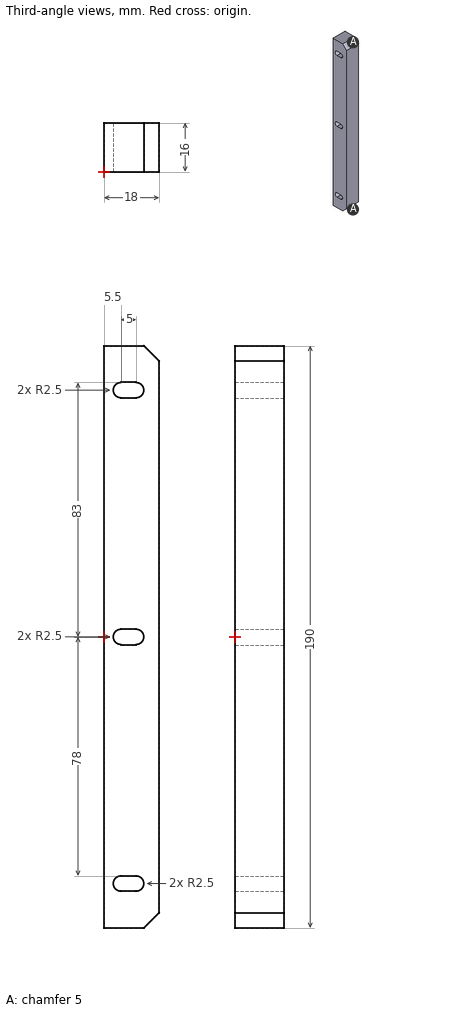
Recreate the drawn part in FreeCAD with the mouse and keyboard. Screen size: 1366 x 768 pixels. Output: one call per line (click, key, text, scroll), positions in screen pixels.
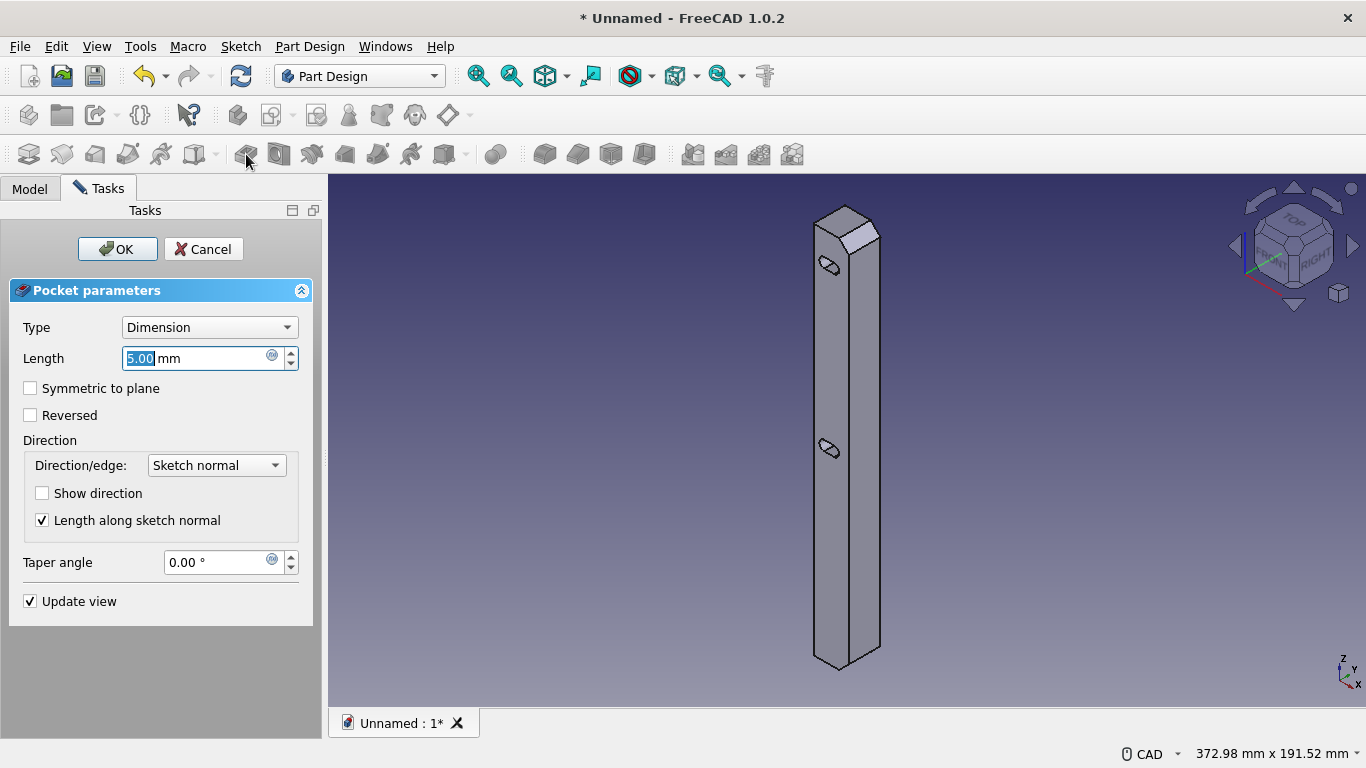
click(210, 328)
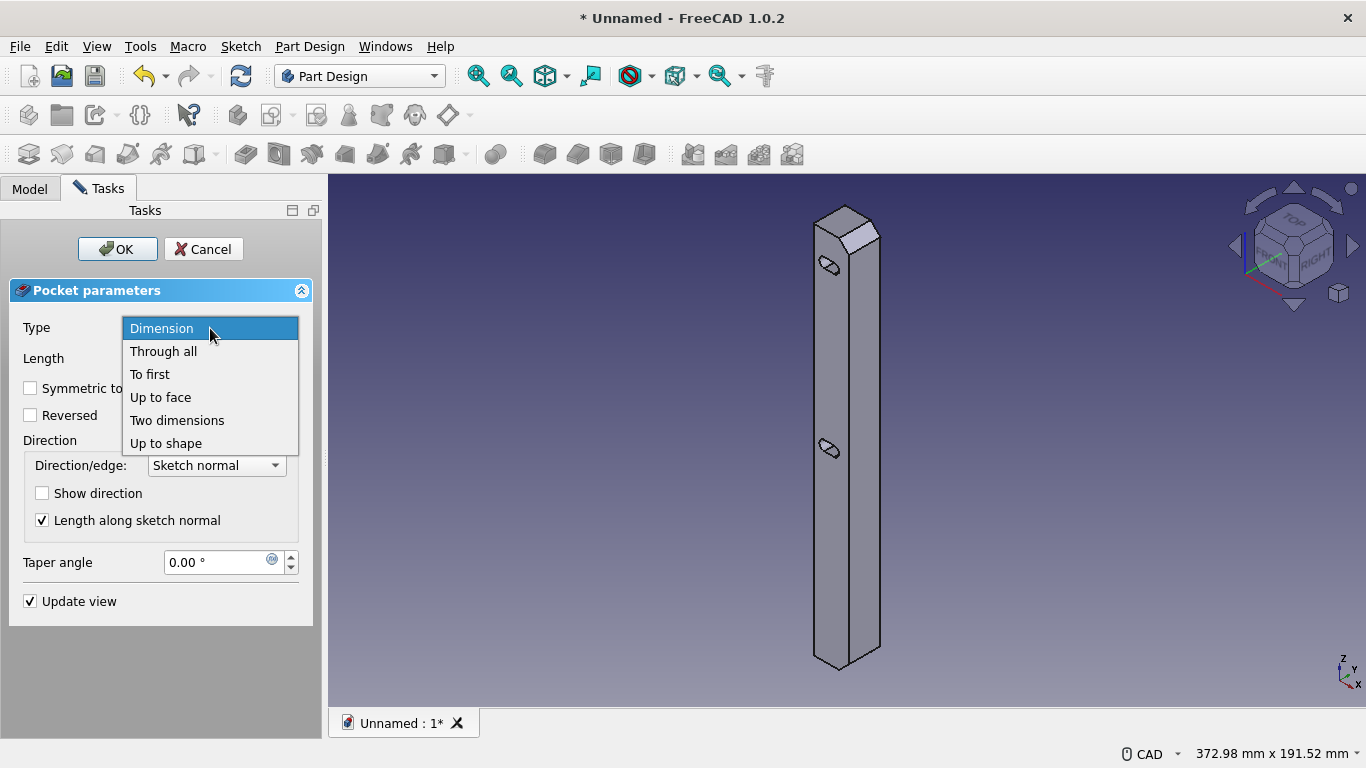
click(208, 374)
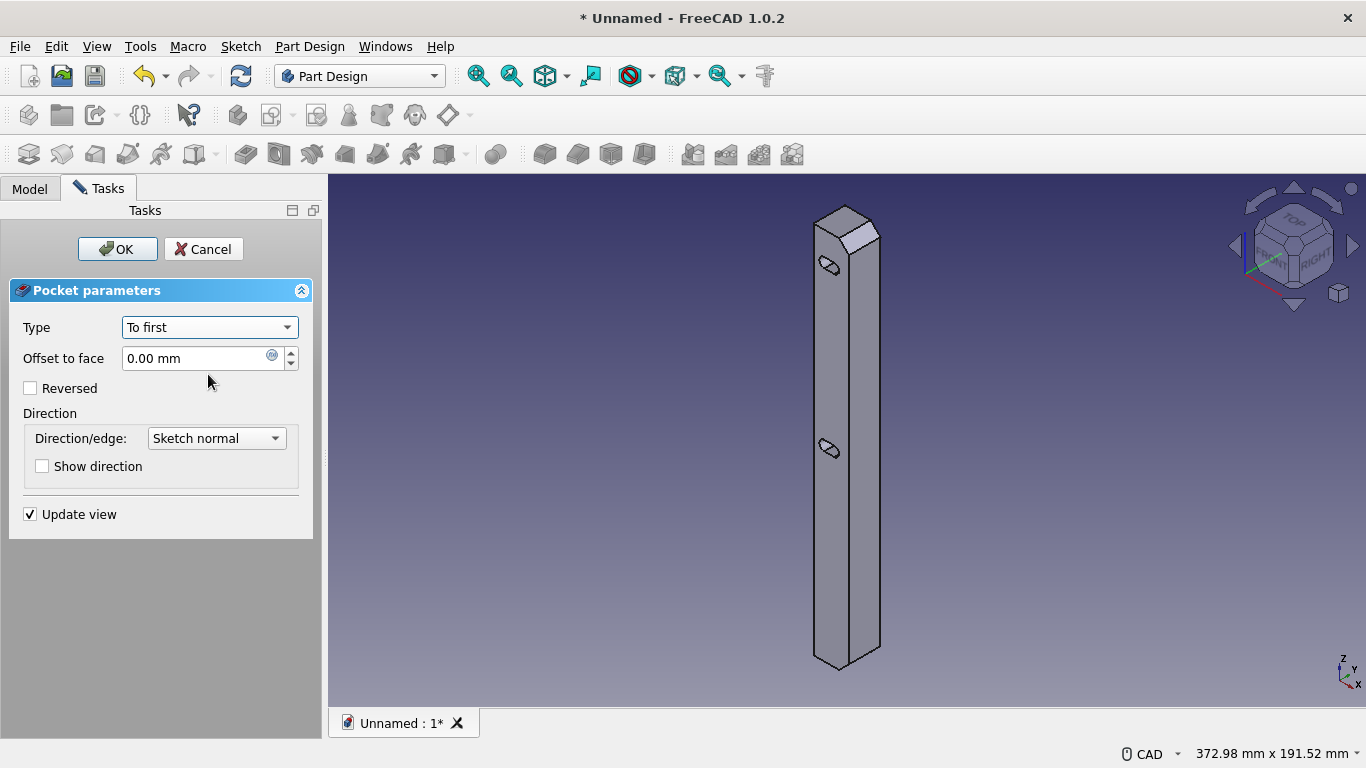
click(118, 249)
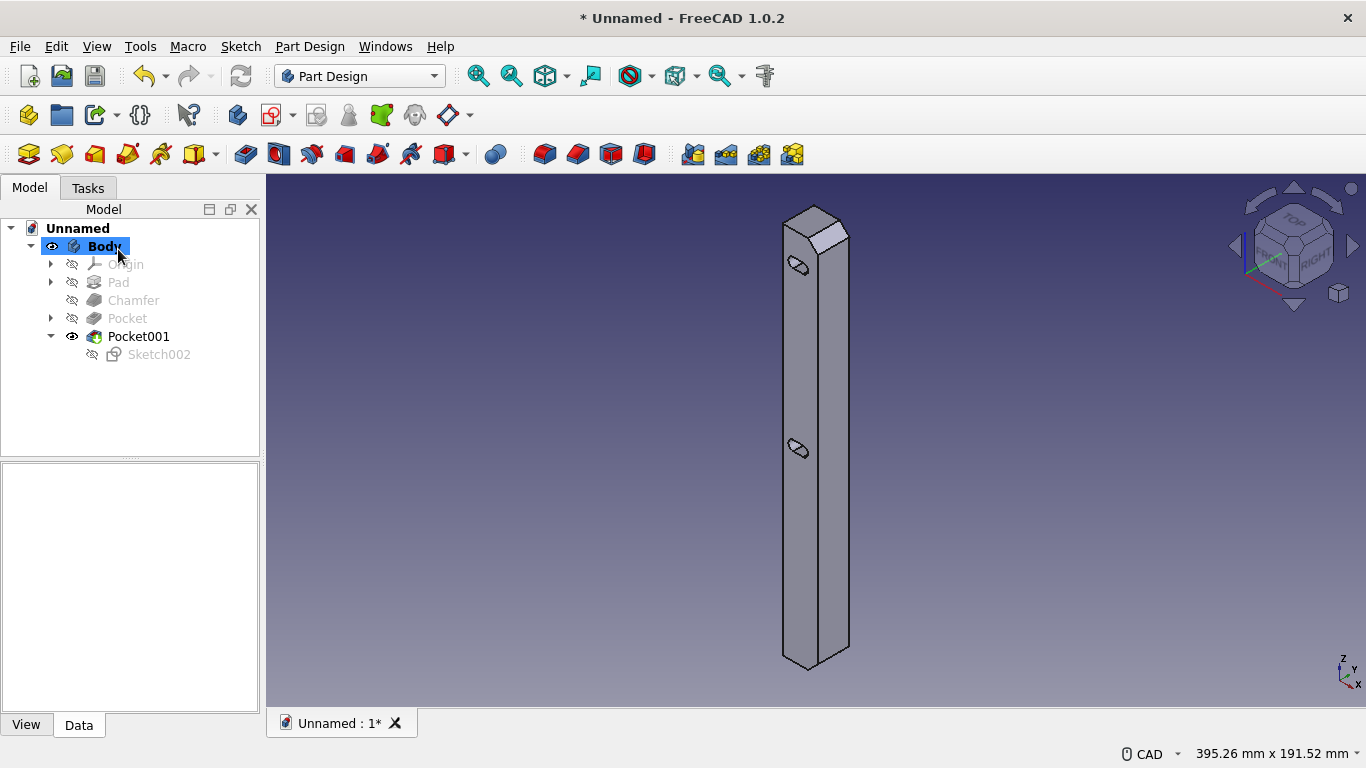
click(800, 325)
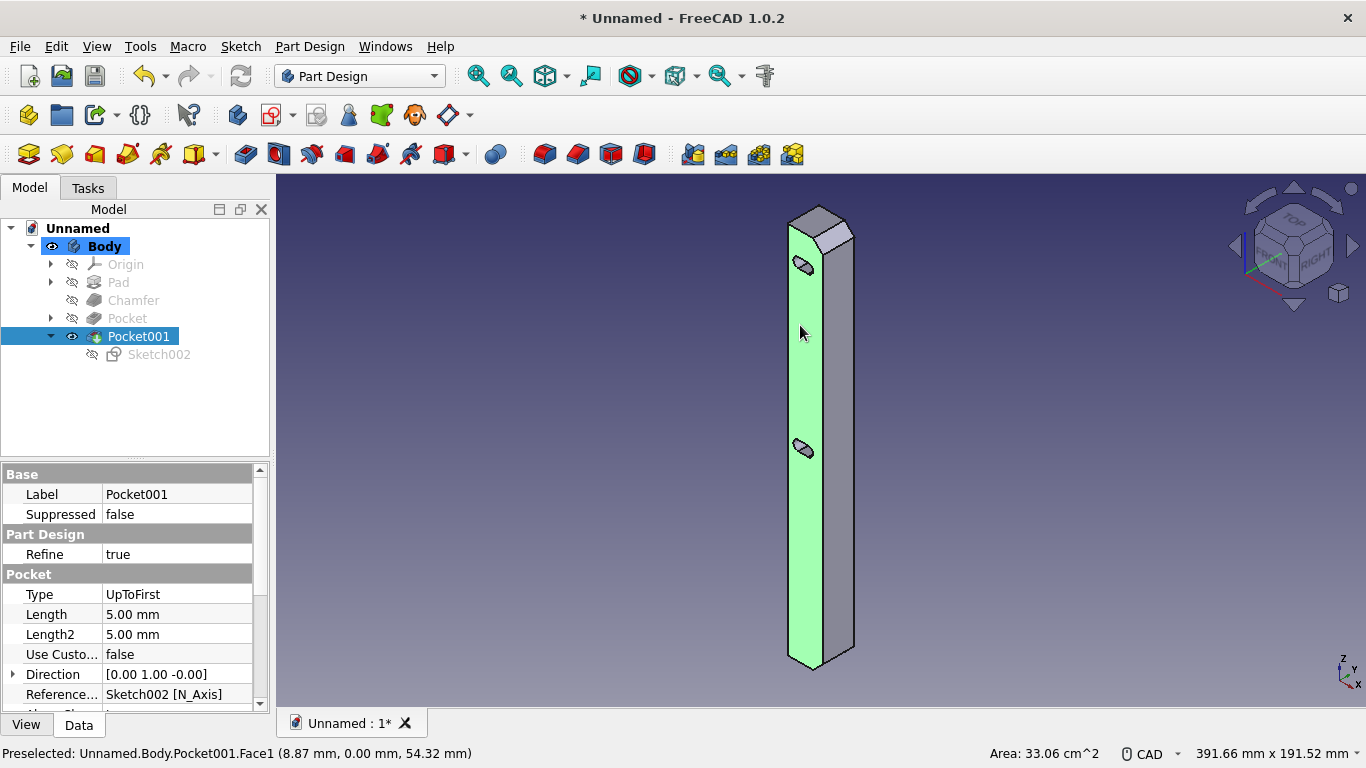
click(270, 116)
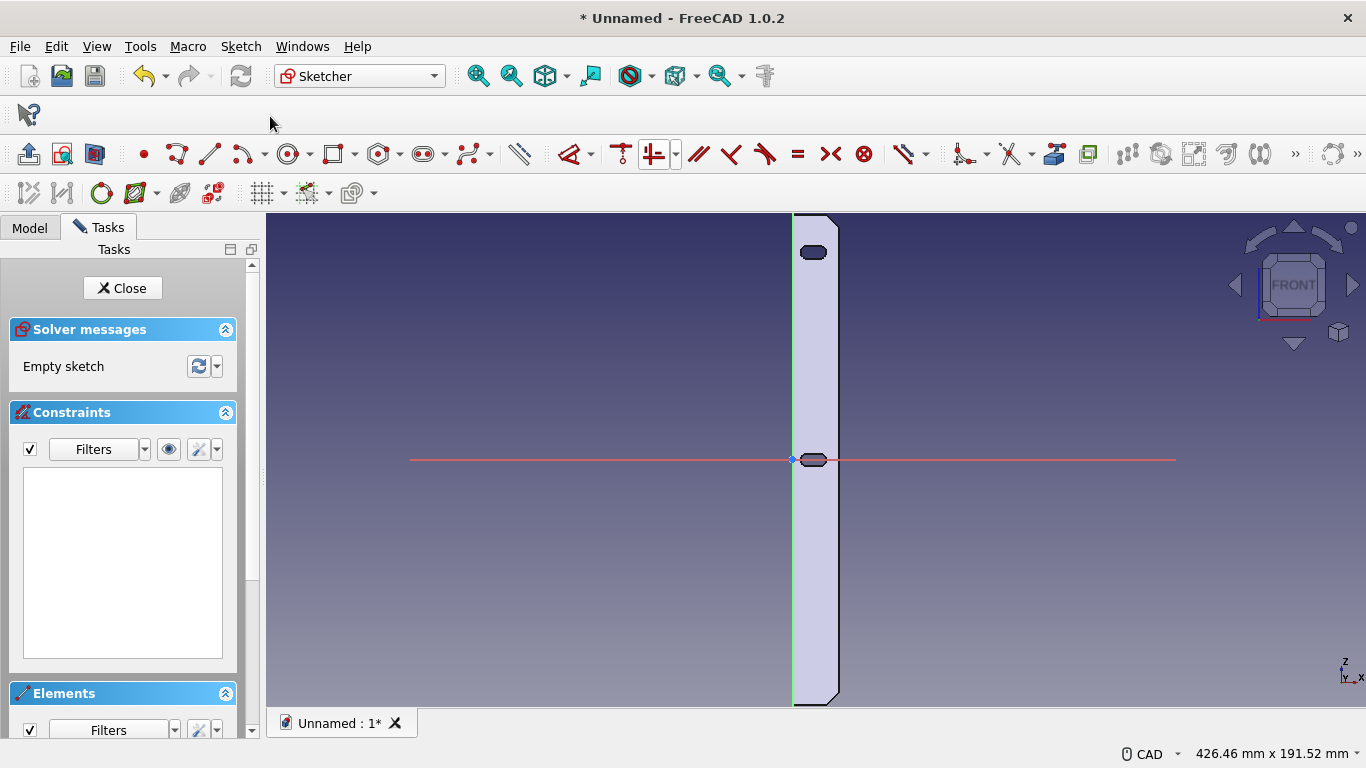
scroll(817, 679, up, 15)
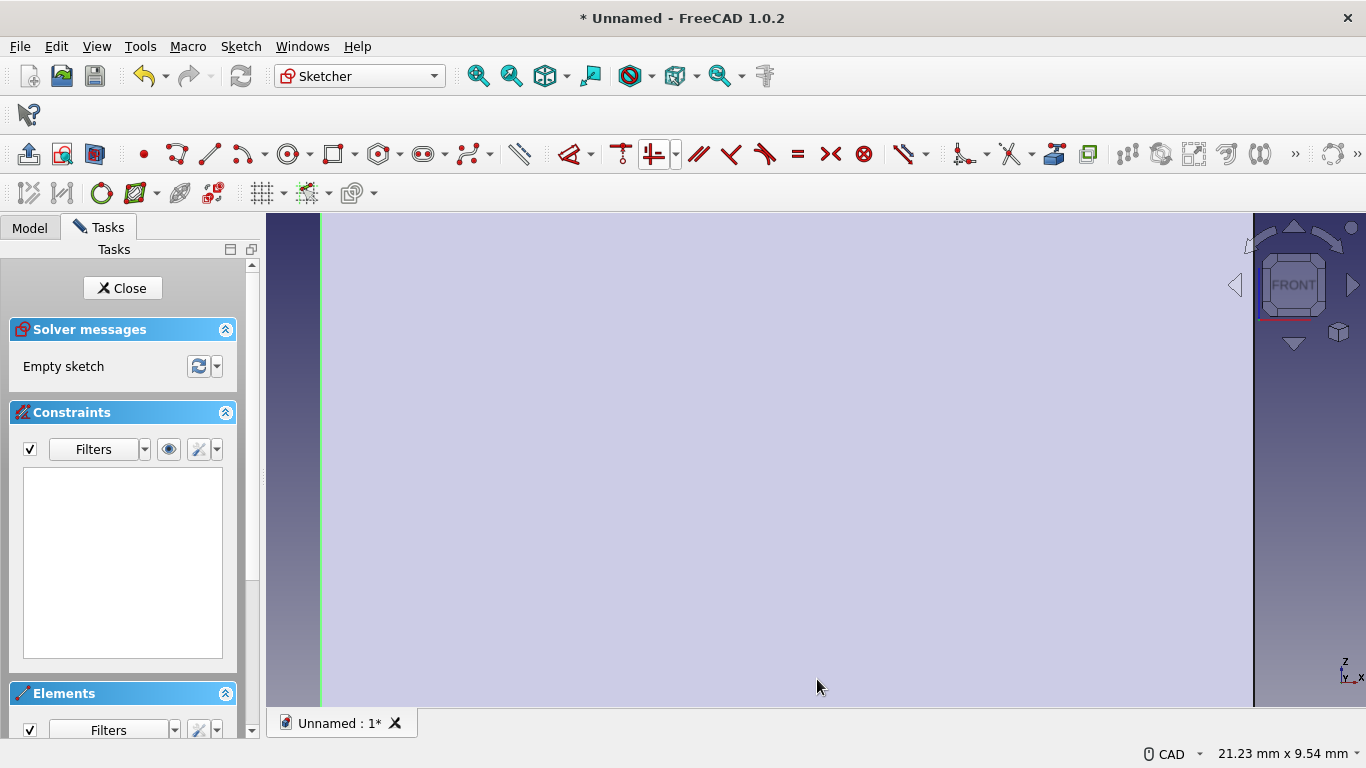
key(g)
key(s)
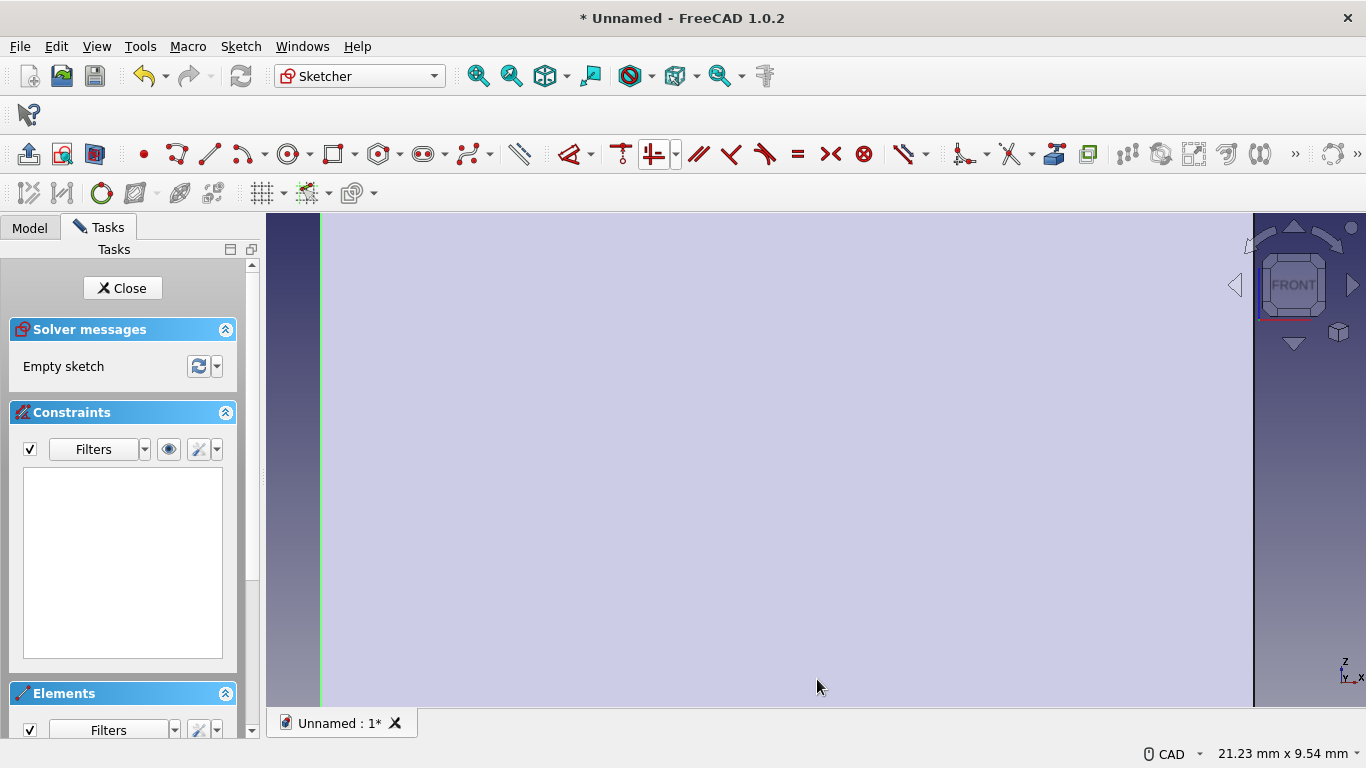
click(606, 433)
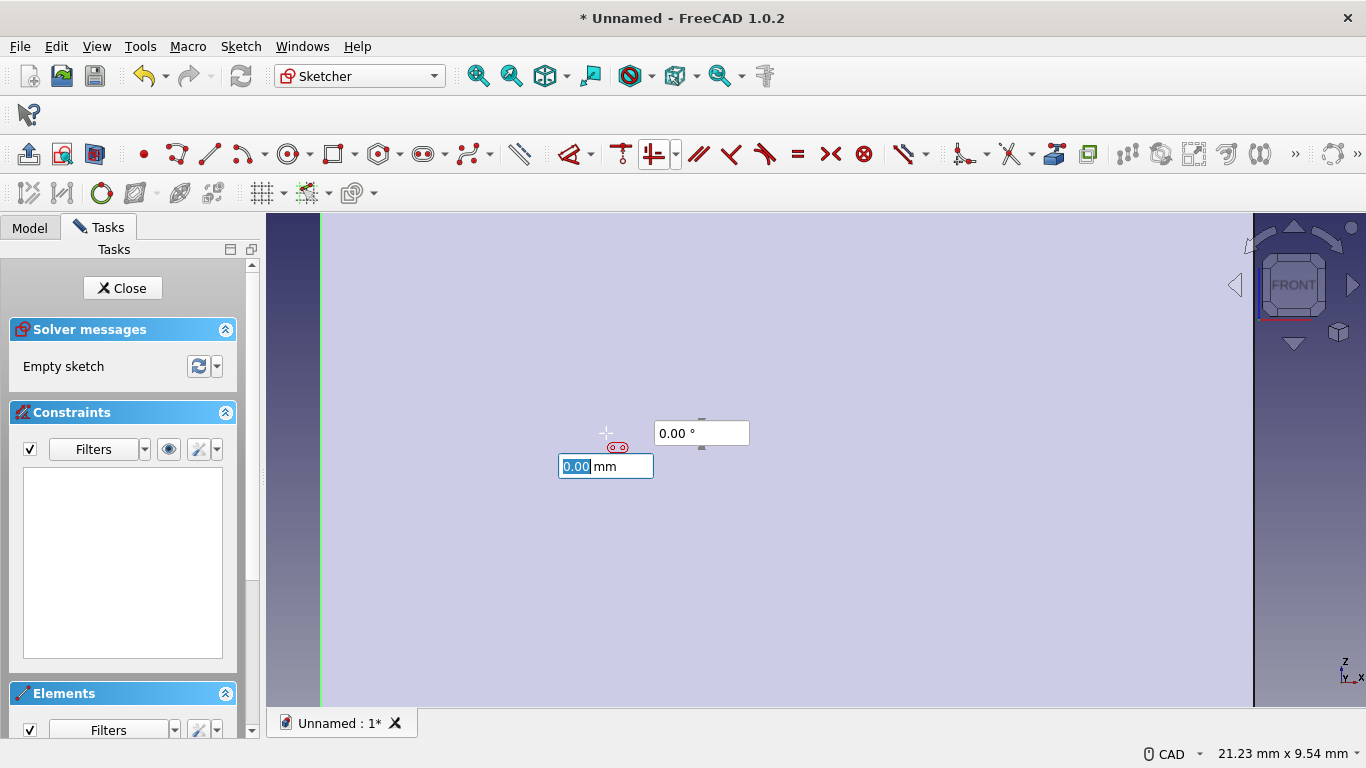
click(865, 433)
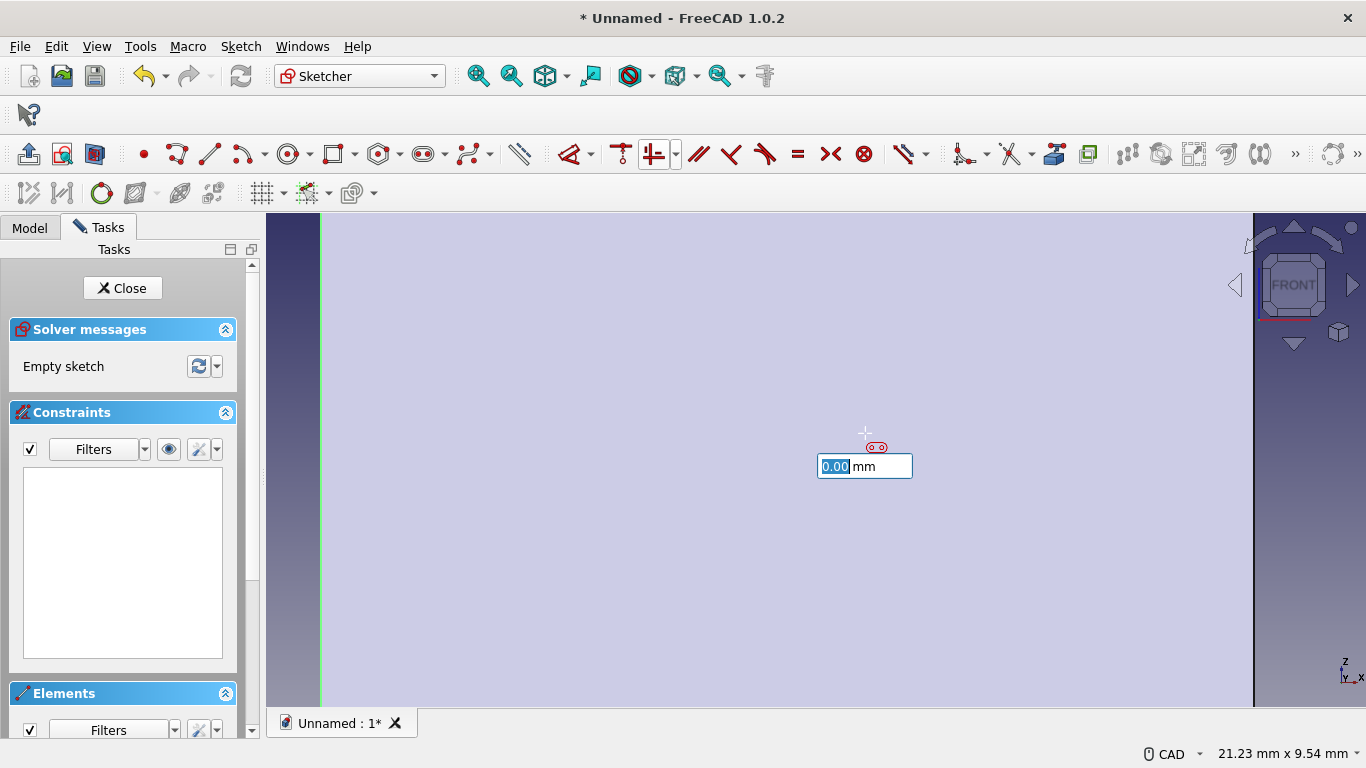
click(736, 562)
key(Escape)